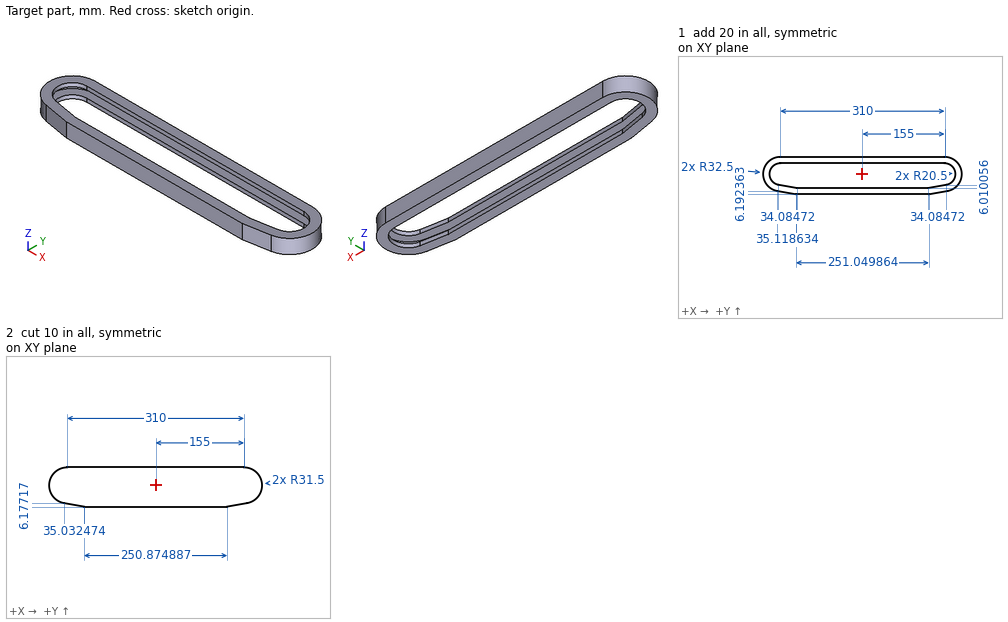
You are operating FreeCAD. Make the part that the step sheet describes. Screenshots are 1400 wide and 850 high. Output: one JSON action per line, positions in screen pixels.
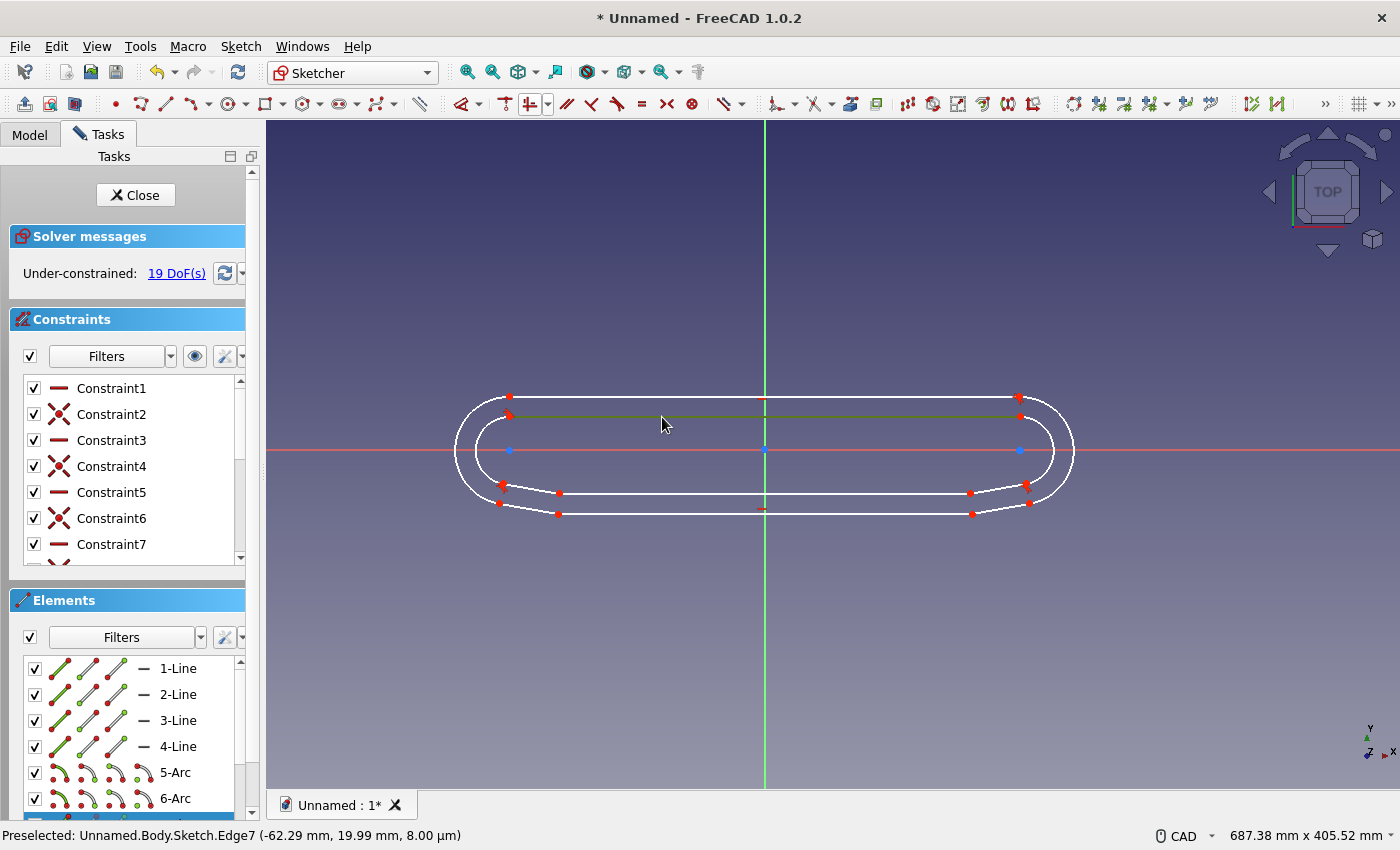
{"action": "left_click", "coordinate": [483, 430]}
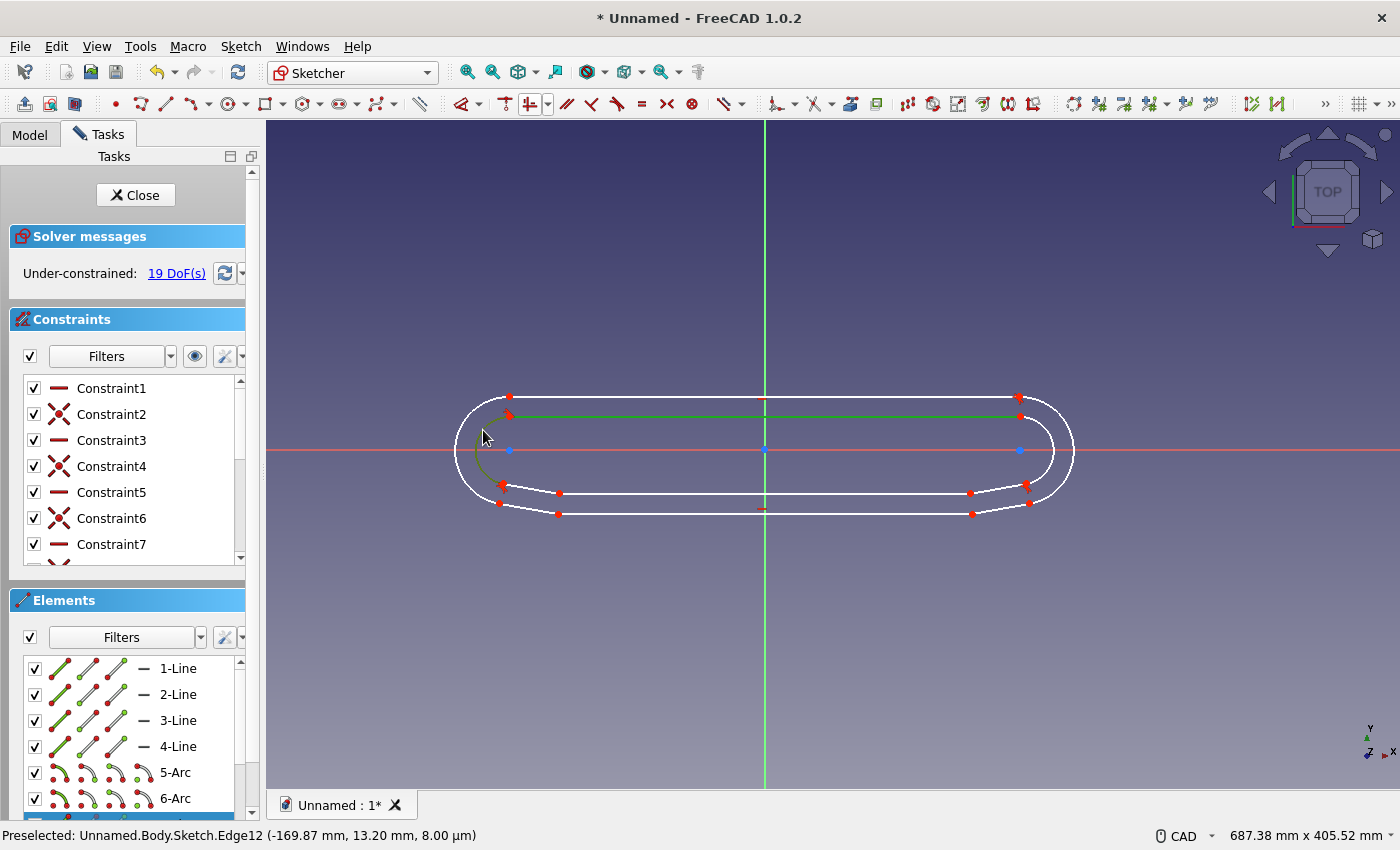
{"action": "left_click", "coordinate": [617, 104]}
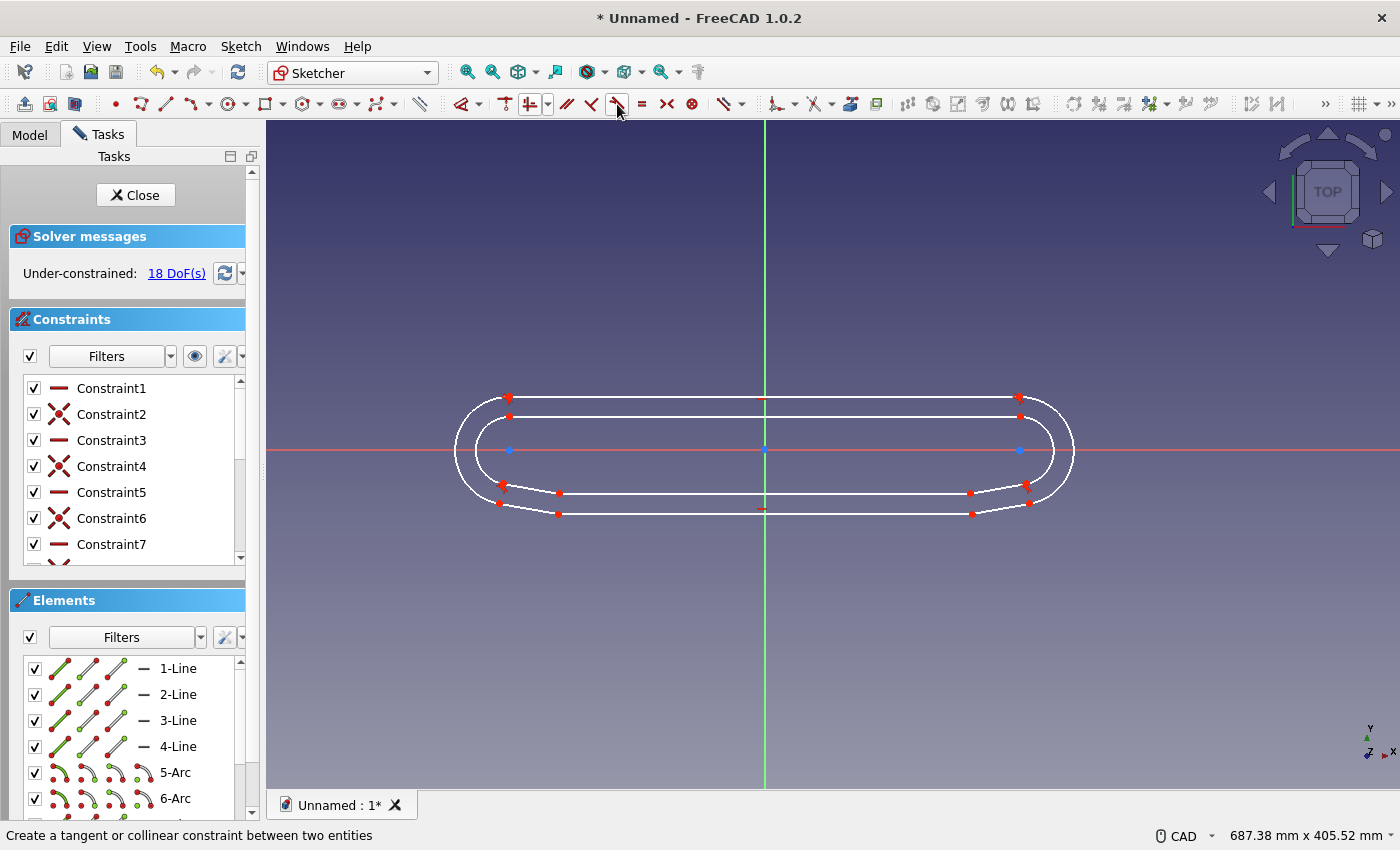
{"action": "left_click", "coordinate": [1009, 487]}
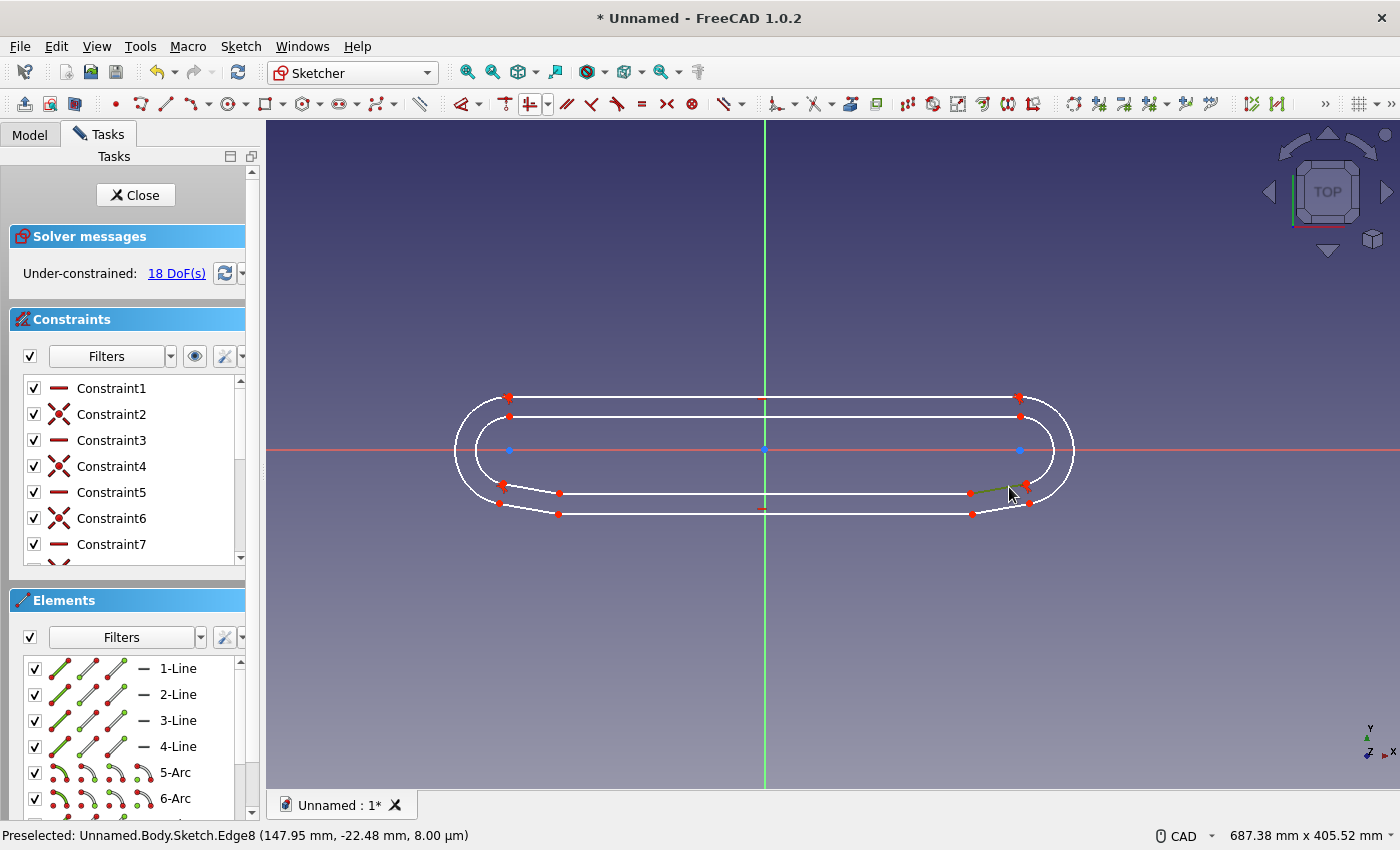
{"action": "left_click", "coordinate": [1050, 467]}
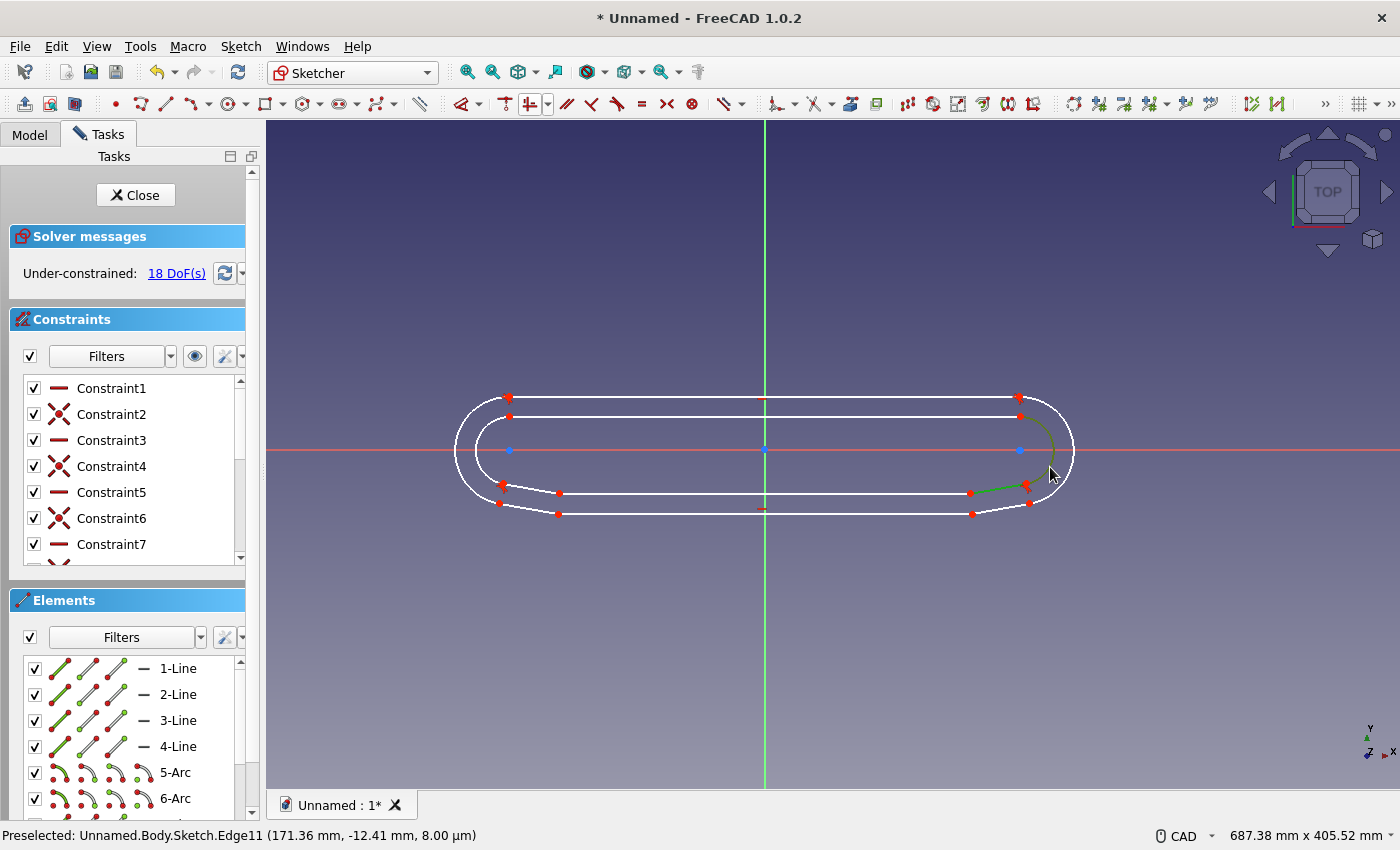
{"action": "key", "text": "t"}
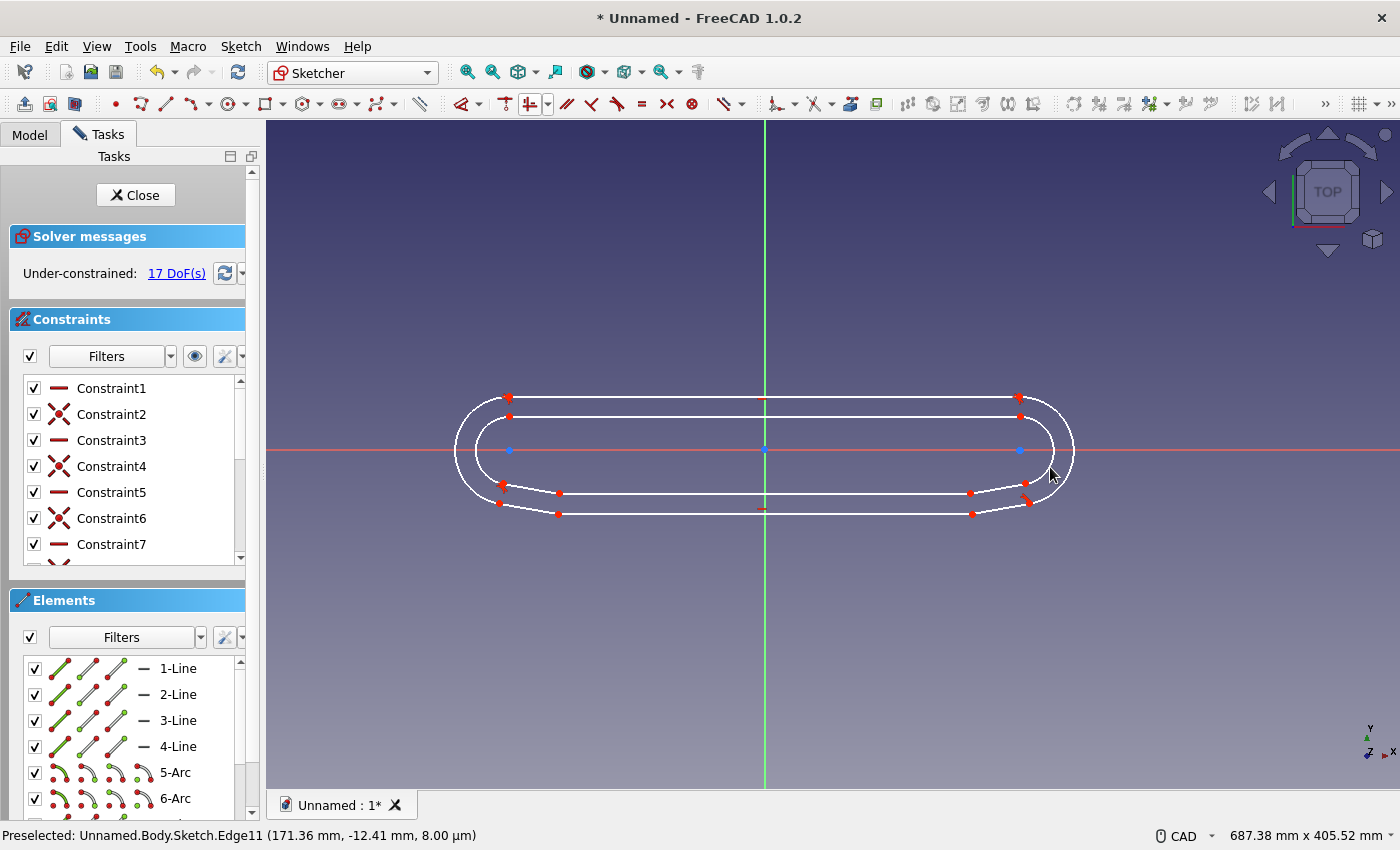
{"action": "left_click", "coordinate": [542, 491]}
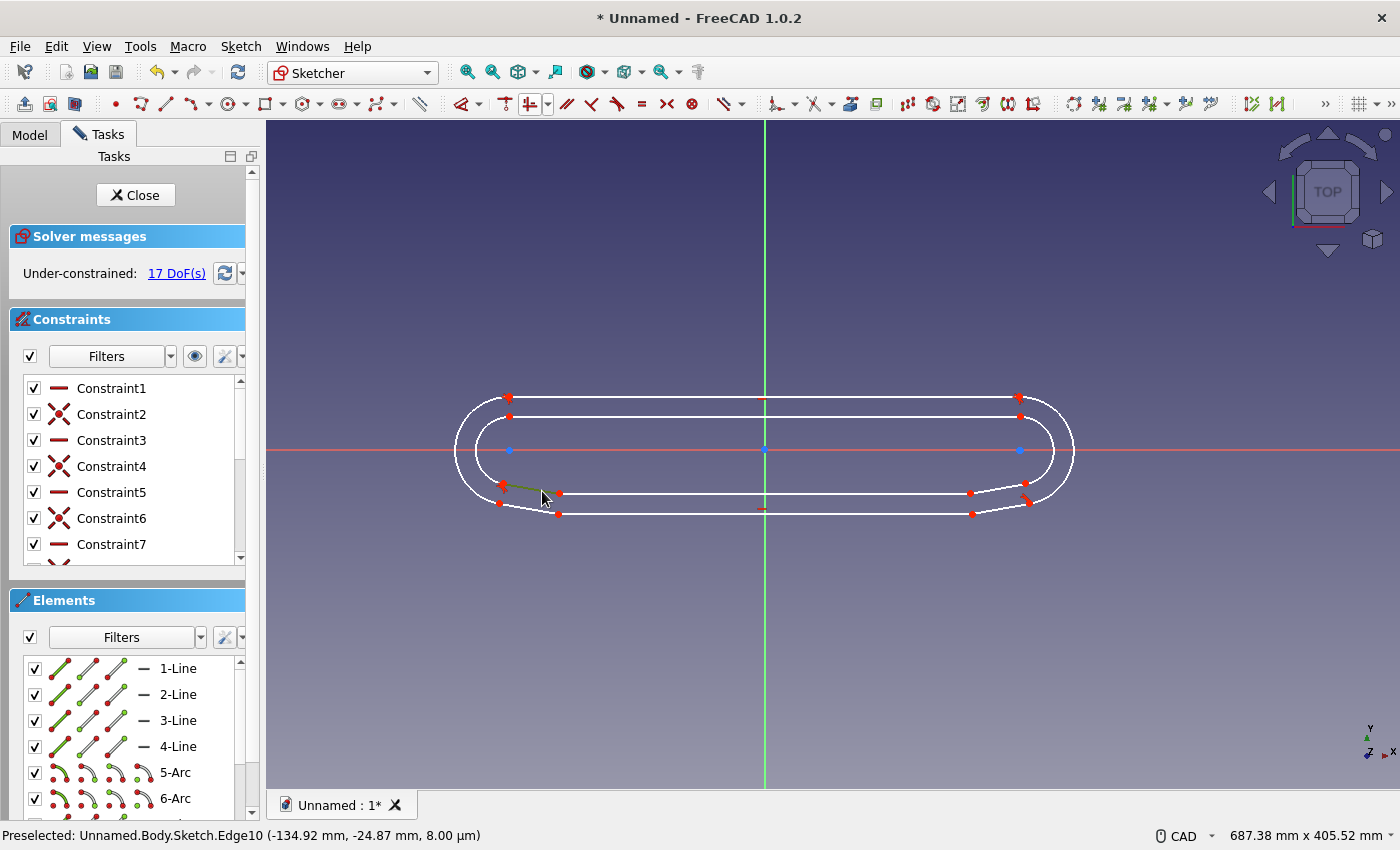
{"action": "left_click", "coordinate": [484, 429]}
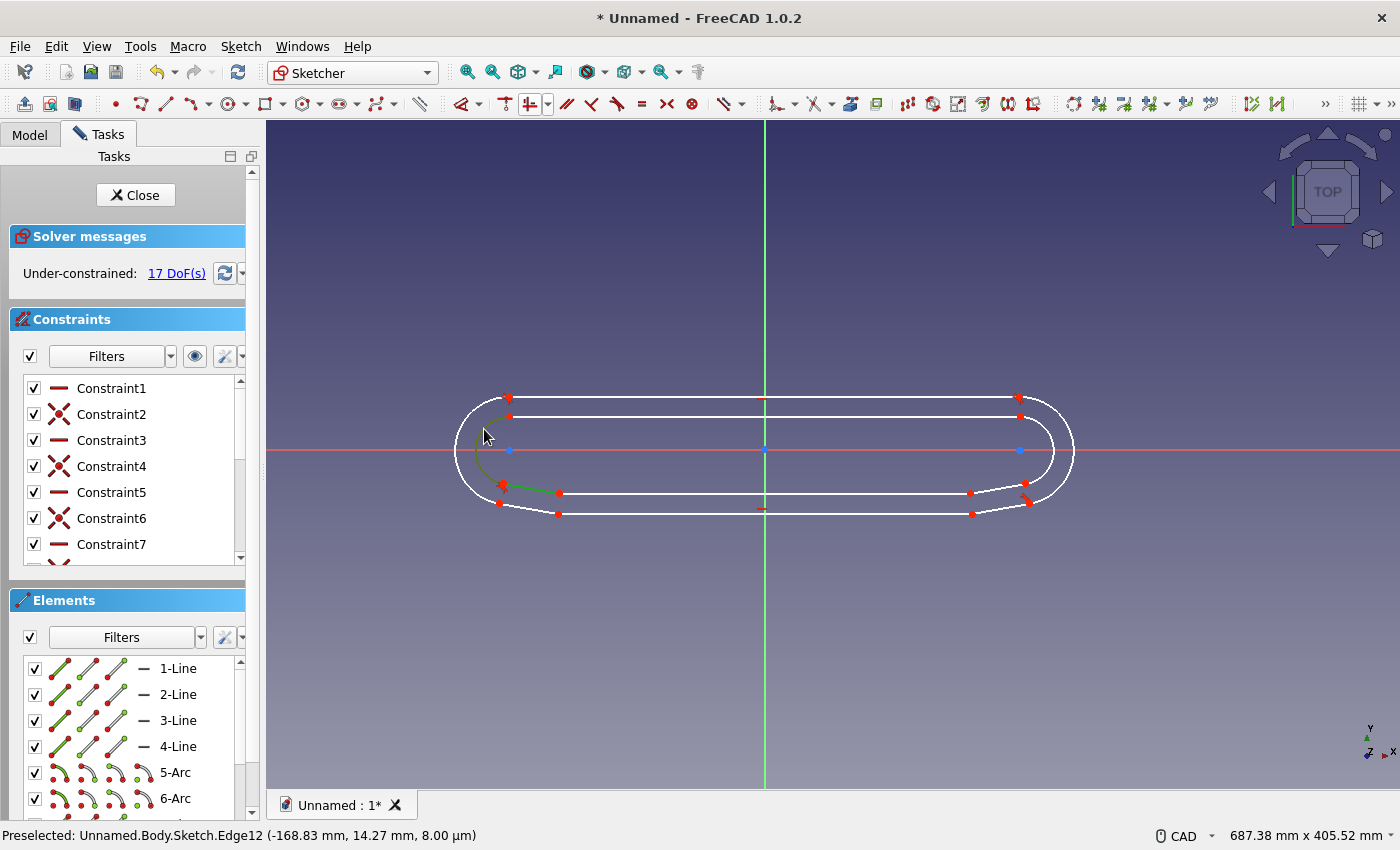
{"action": "key", "text": "t"}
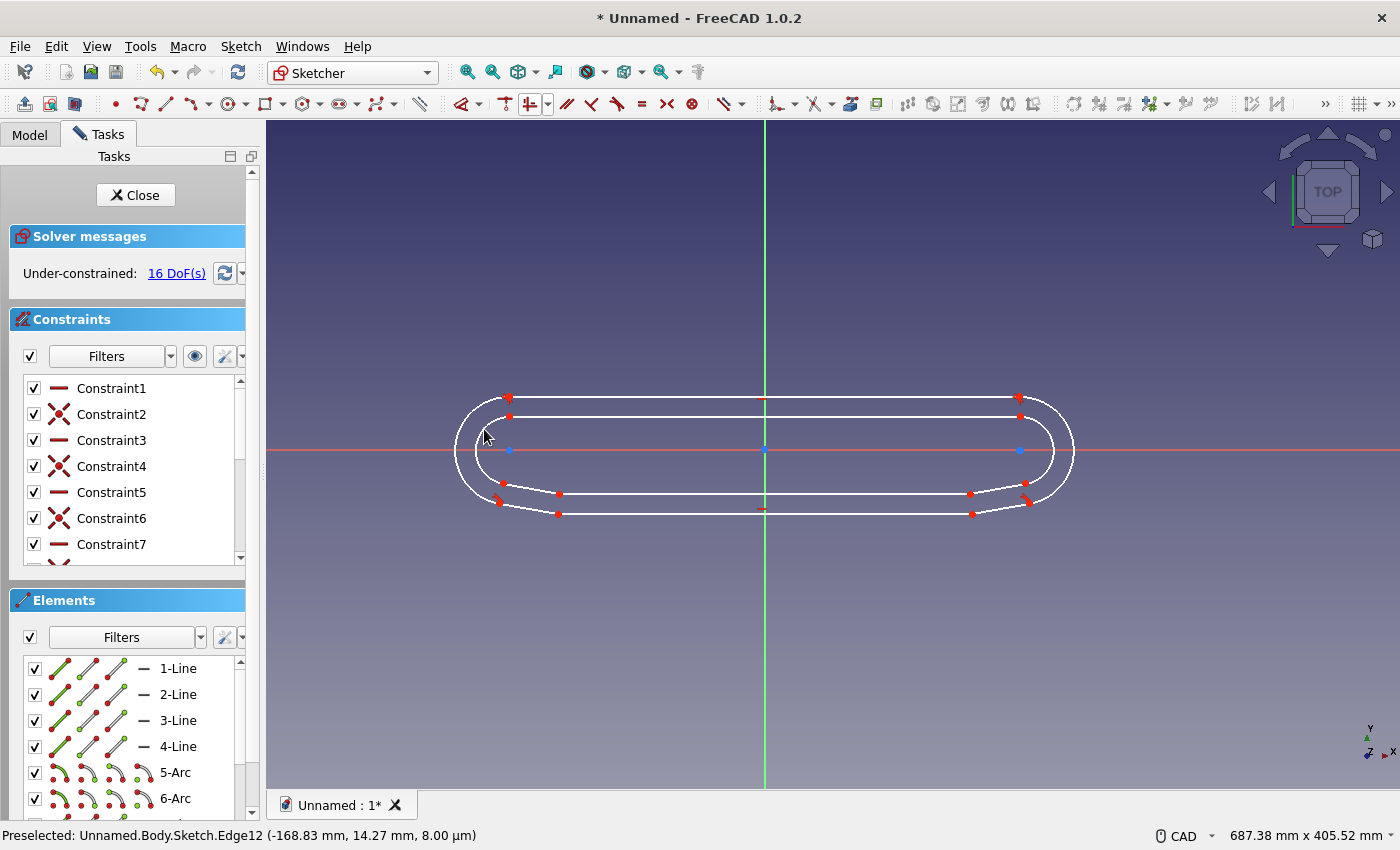
{"action": "left_click", "coordinate": [1067, 477]}